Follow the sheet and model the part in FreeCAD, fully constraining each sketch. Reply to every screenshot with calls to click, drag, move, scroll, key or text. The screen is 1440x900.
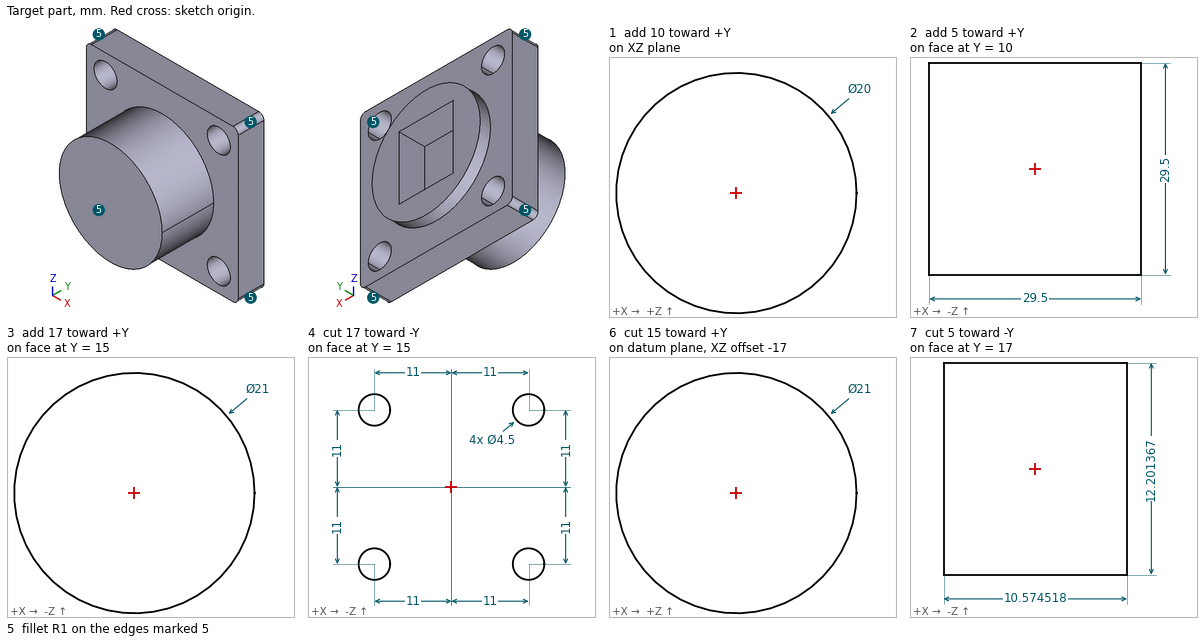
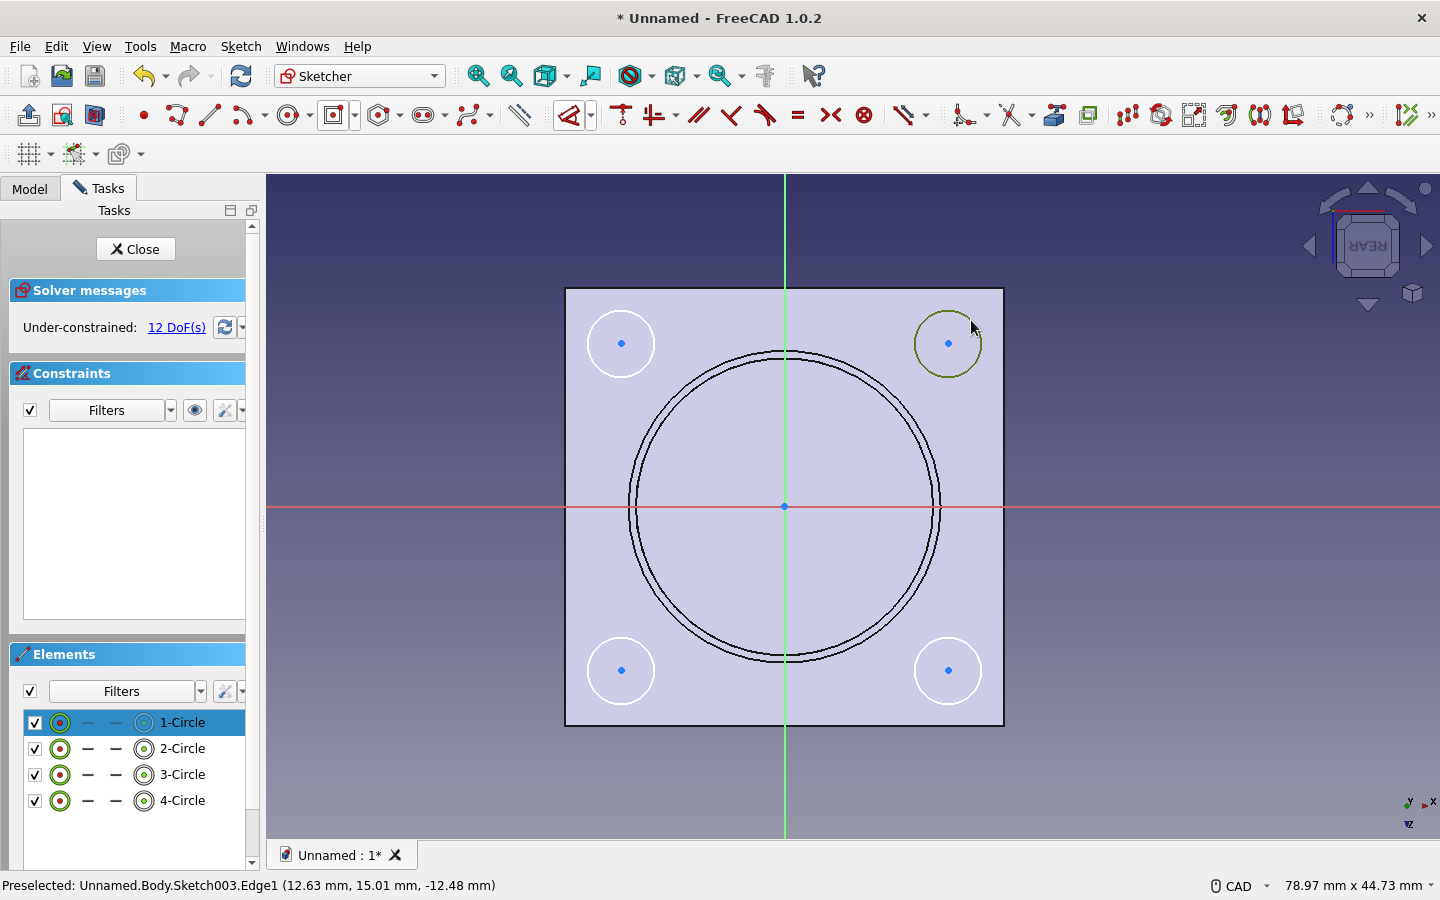
click(644, 320)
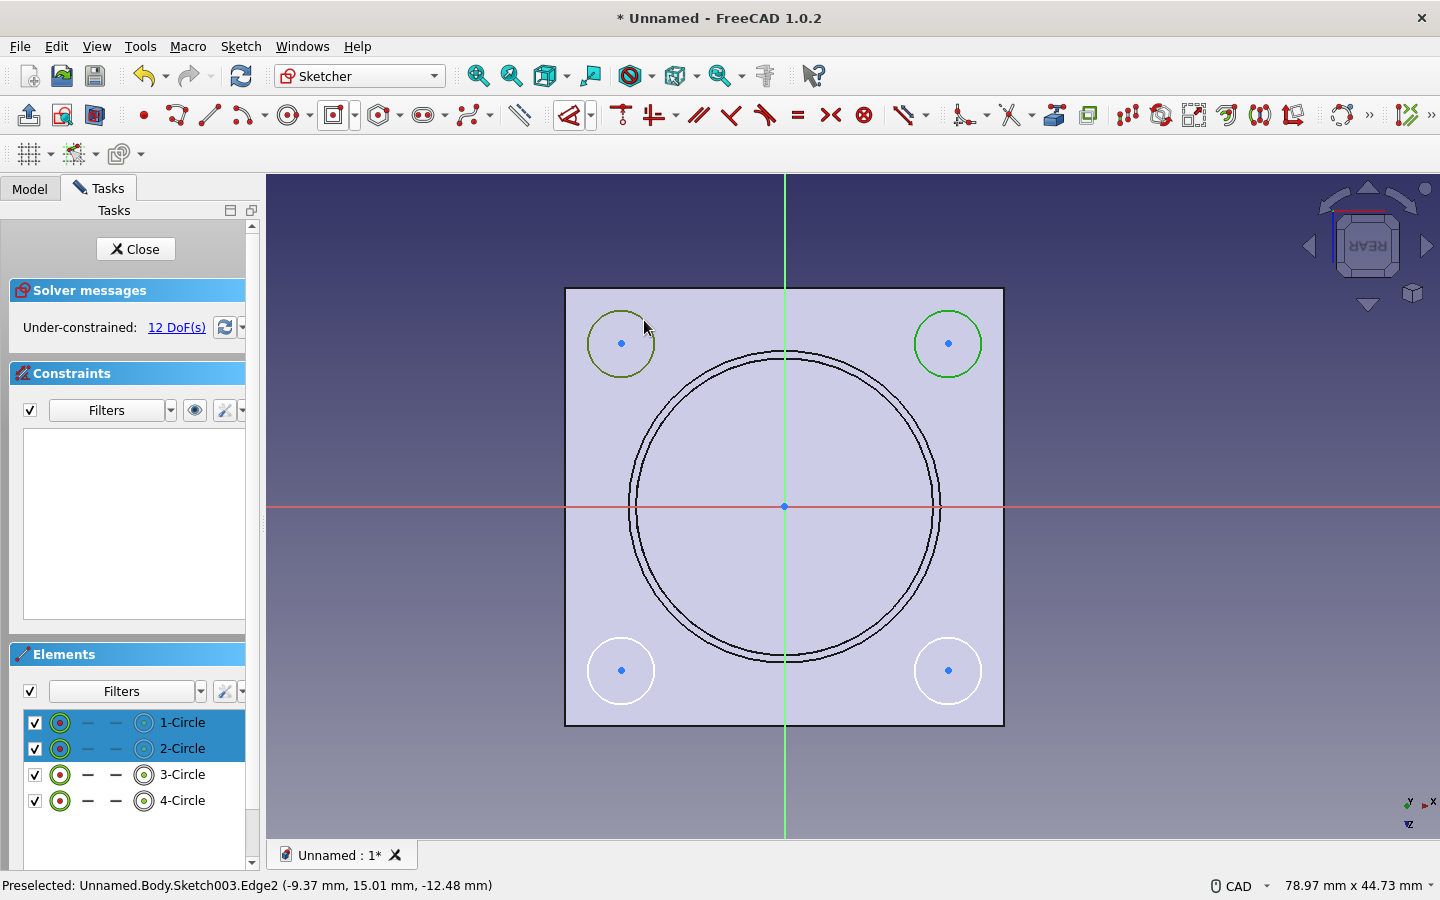
click(644, 647)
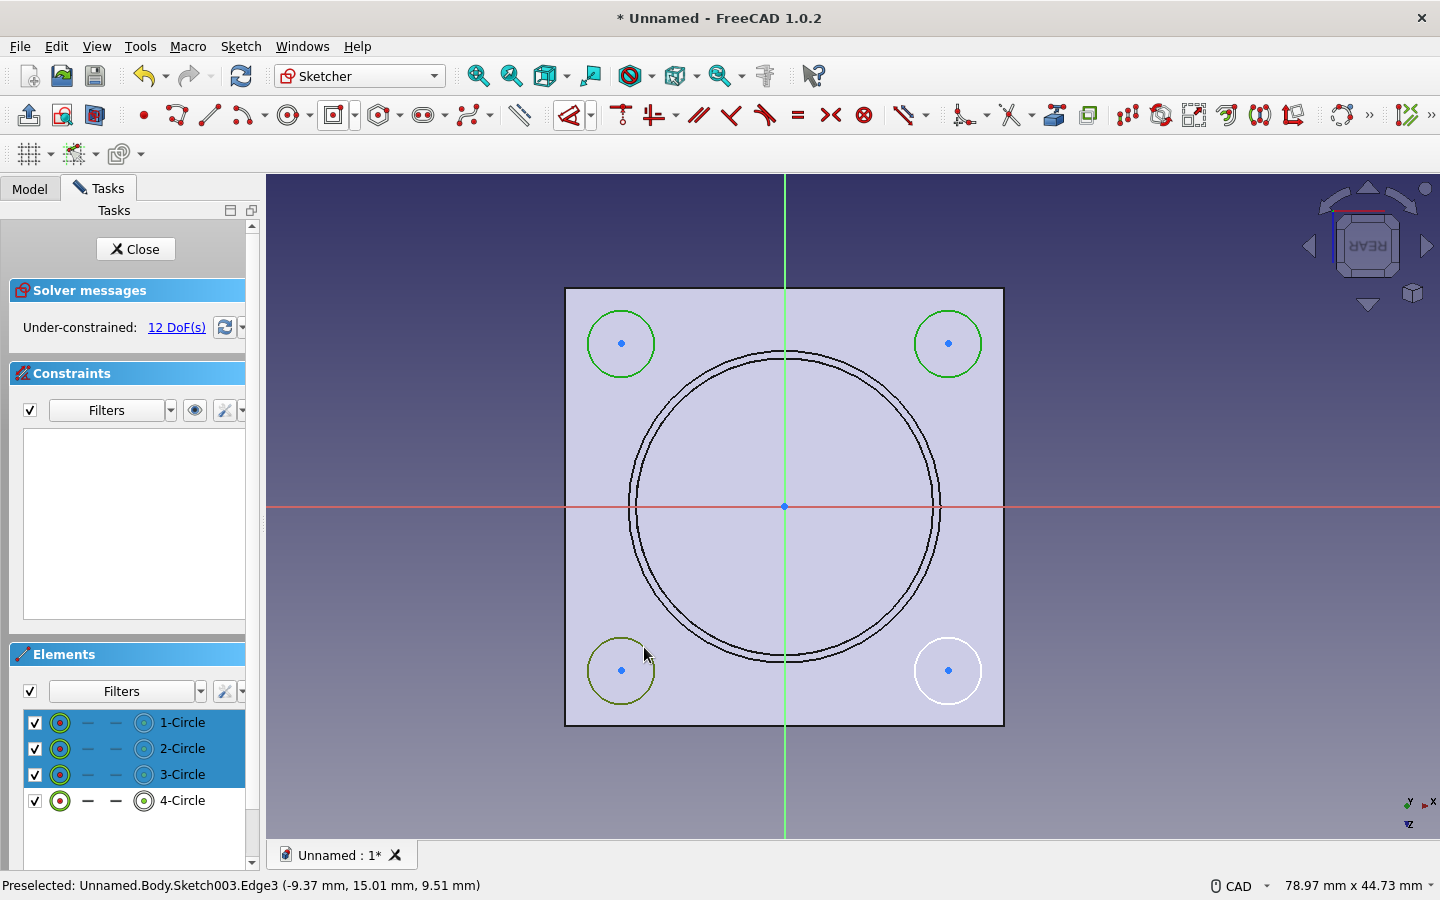
click(971, 647)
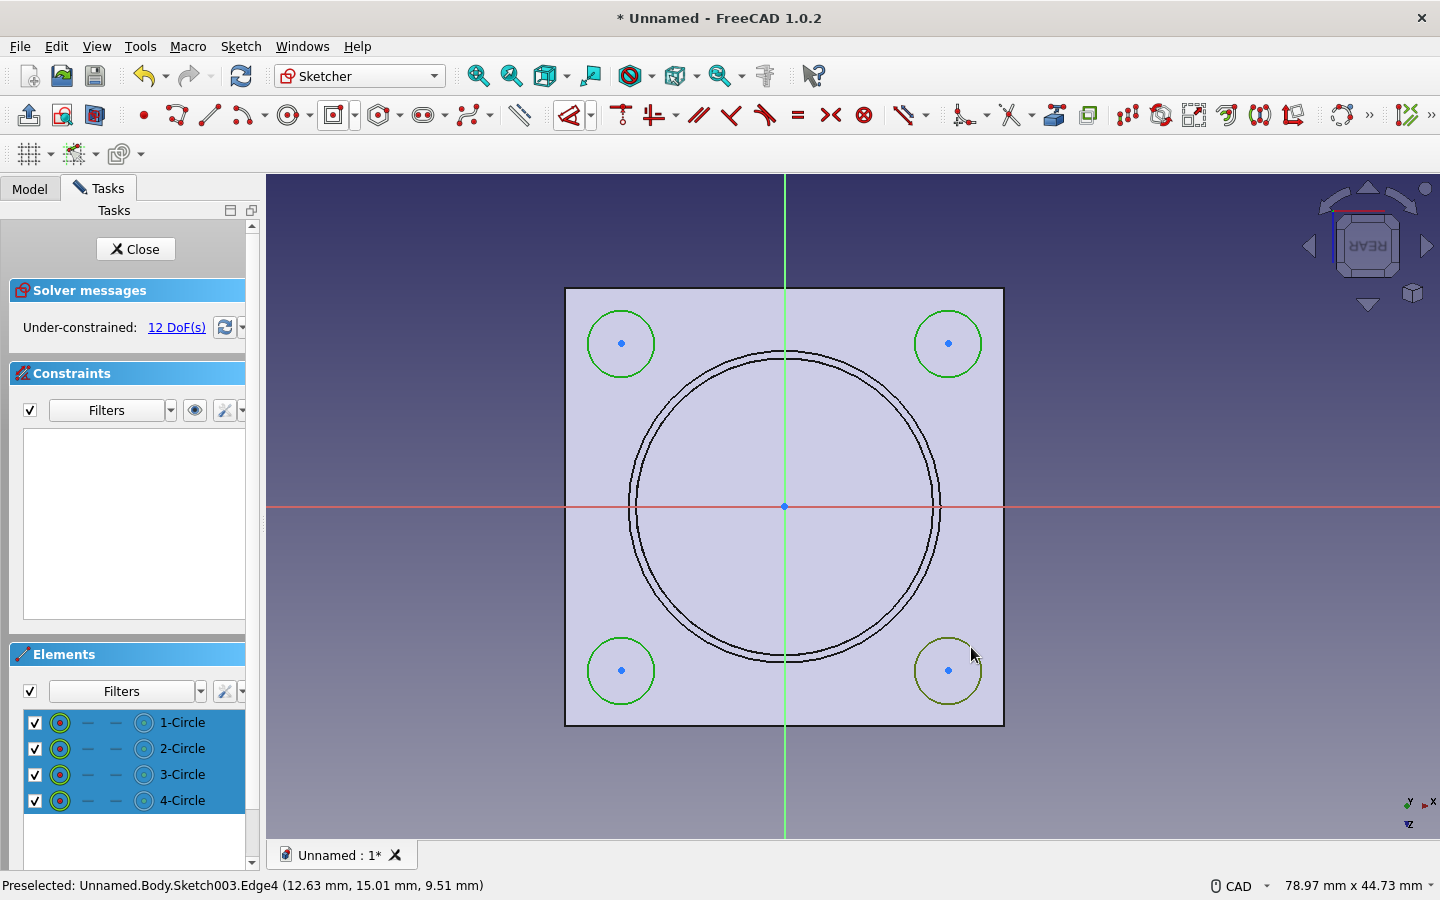
click(798, 116)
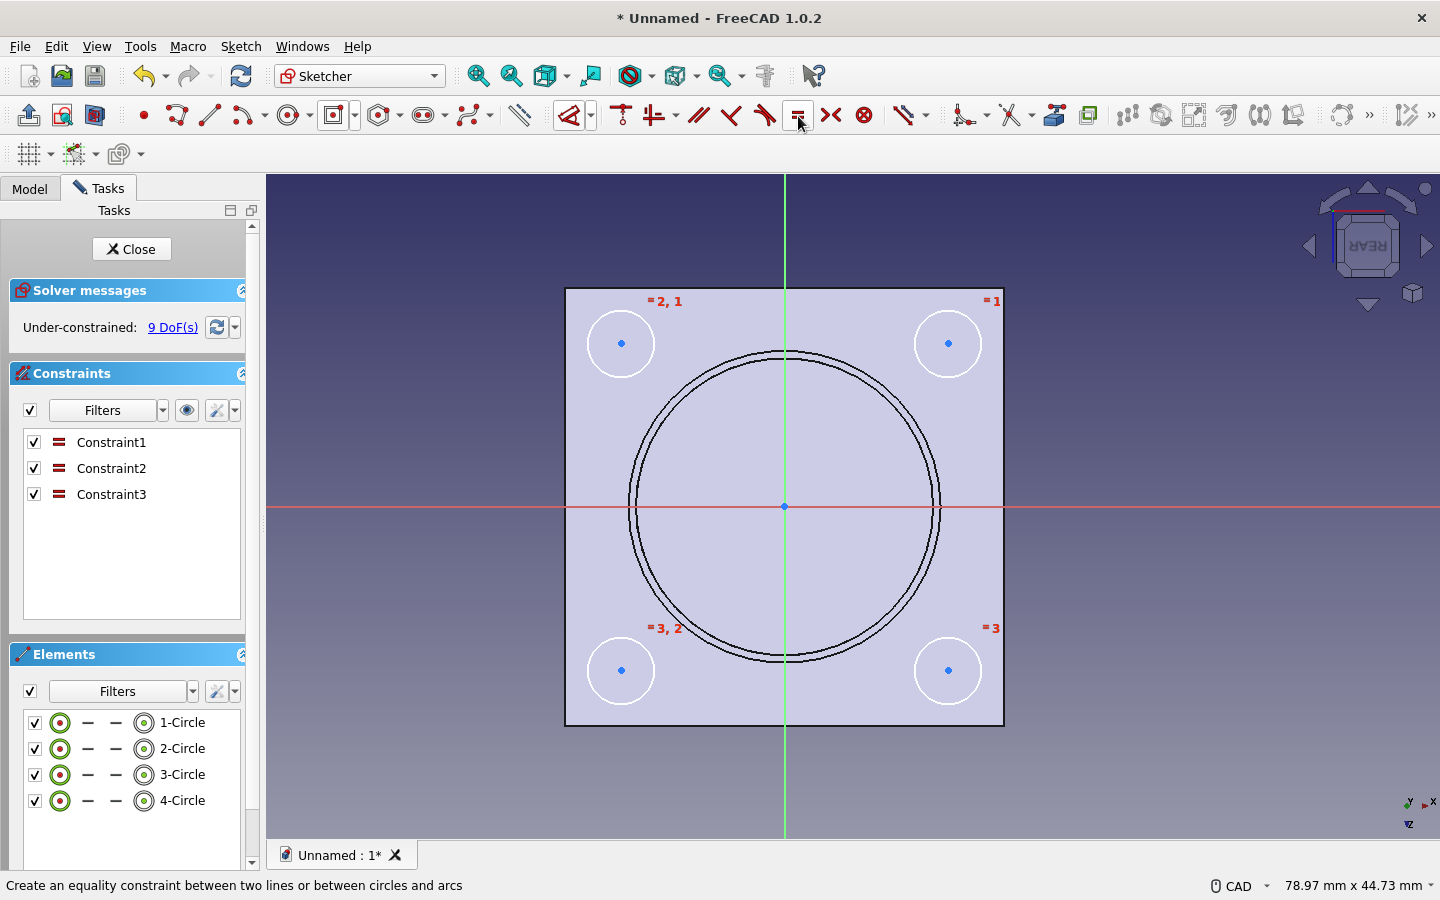
click(971, 320)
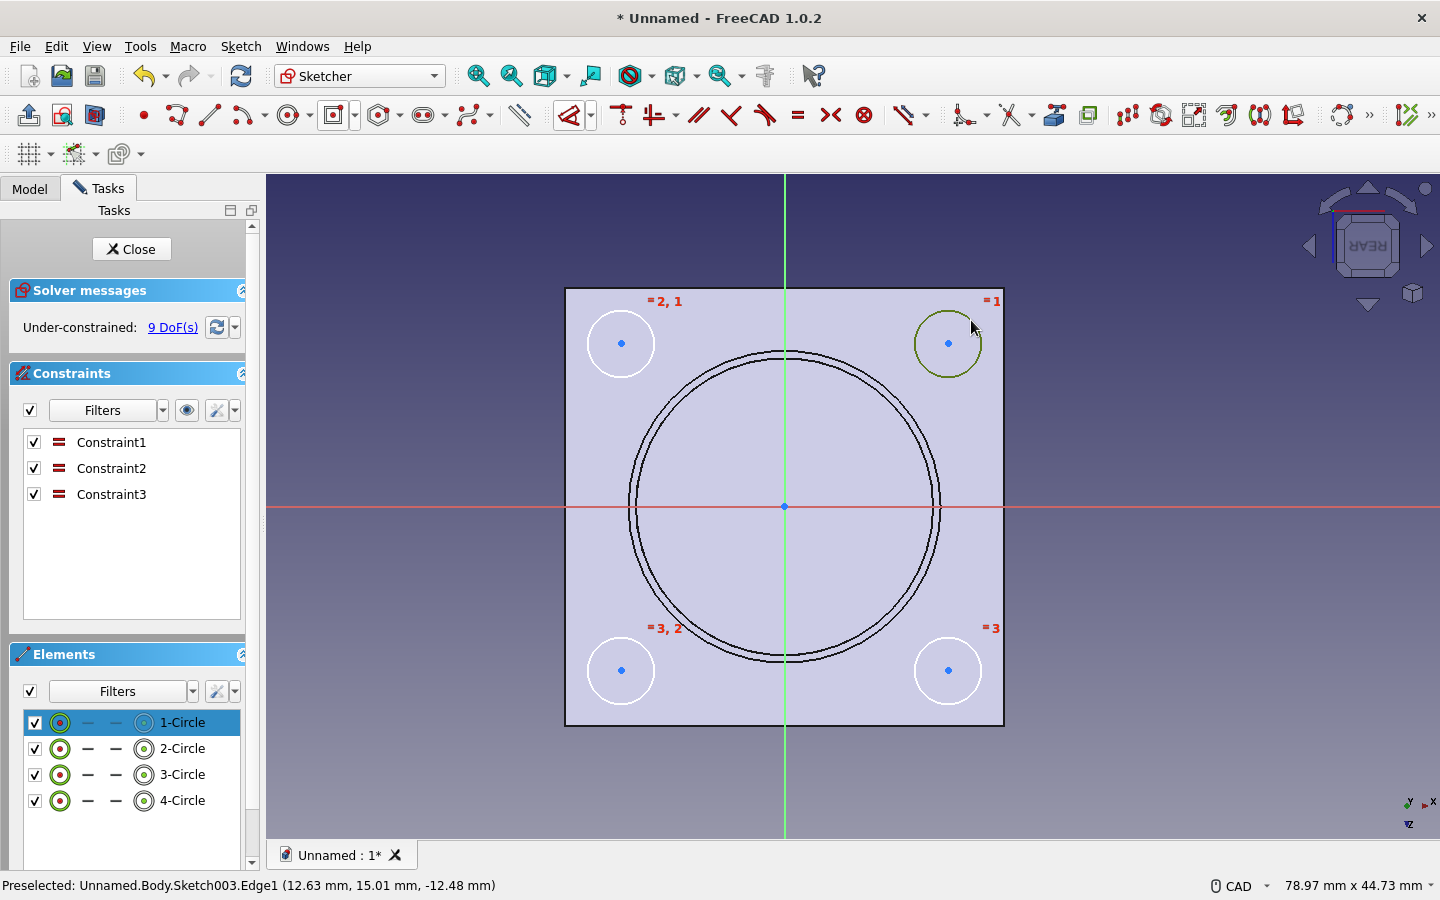
click(590, 116)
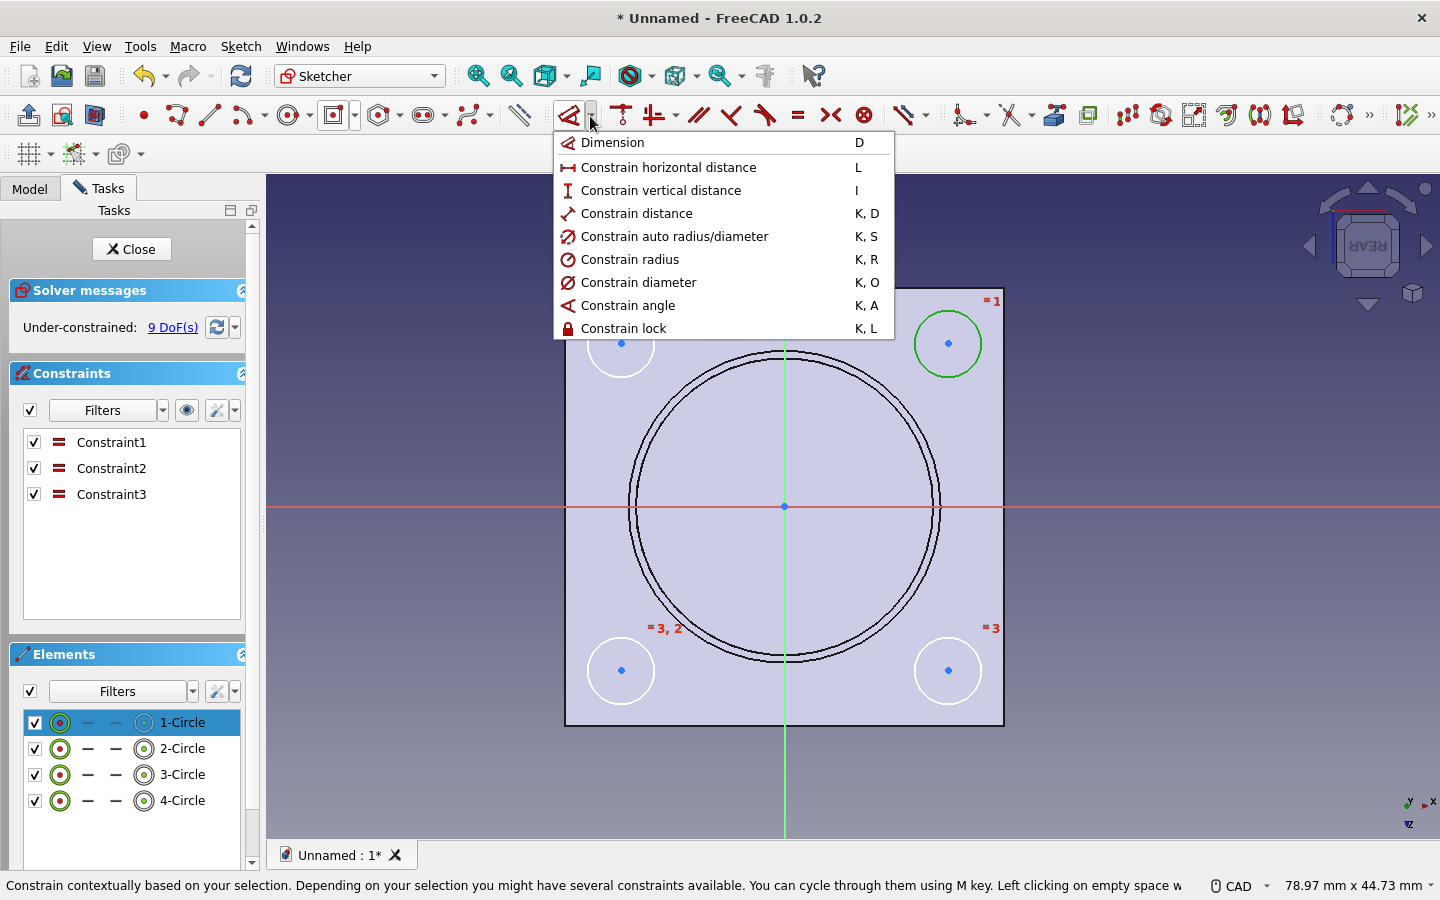
click(724, 282)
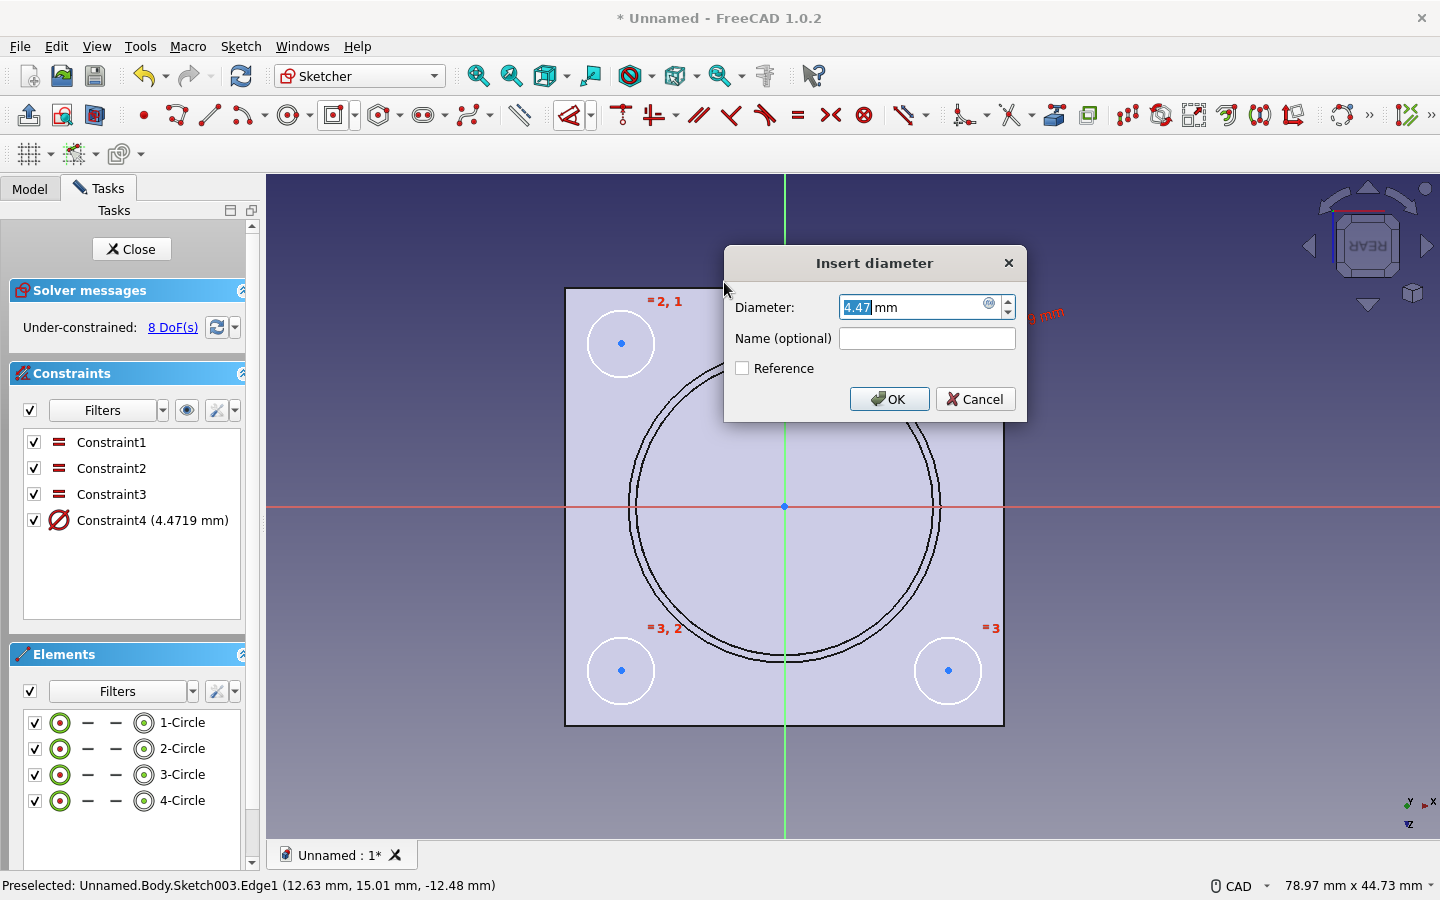
text(4.5)
key(Return)